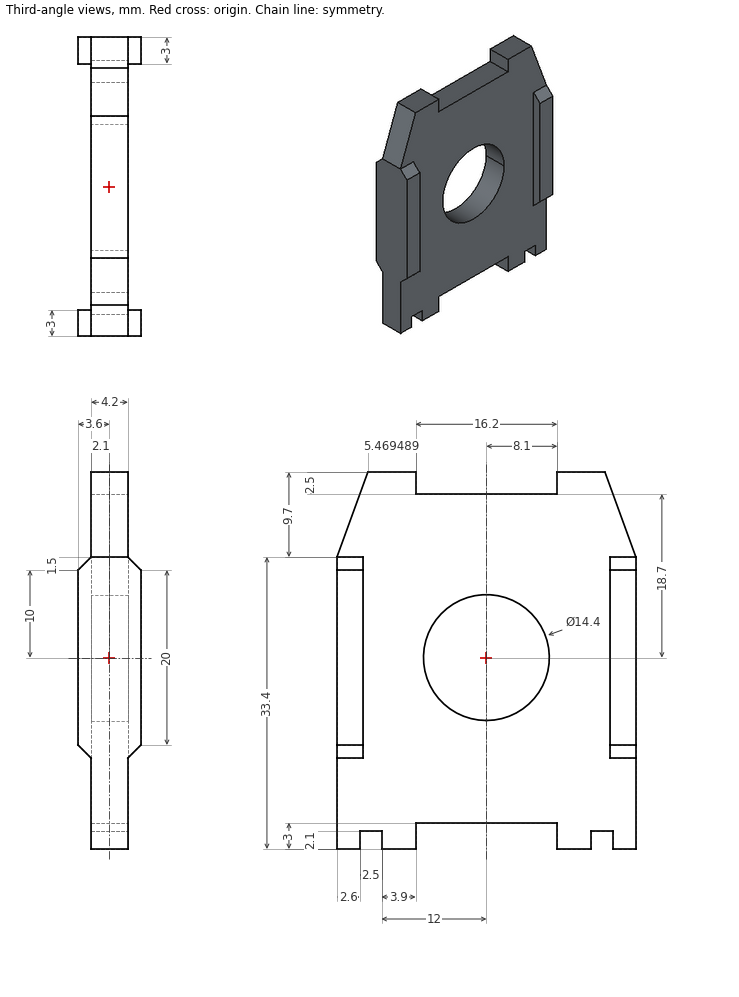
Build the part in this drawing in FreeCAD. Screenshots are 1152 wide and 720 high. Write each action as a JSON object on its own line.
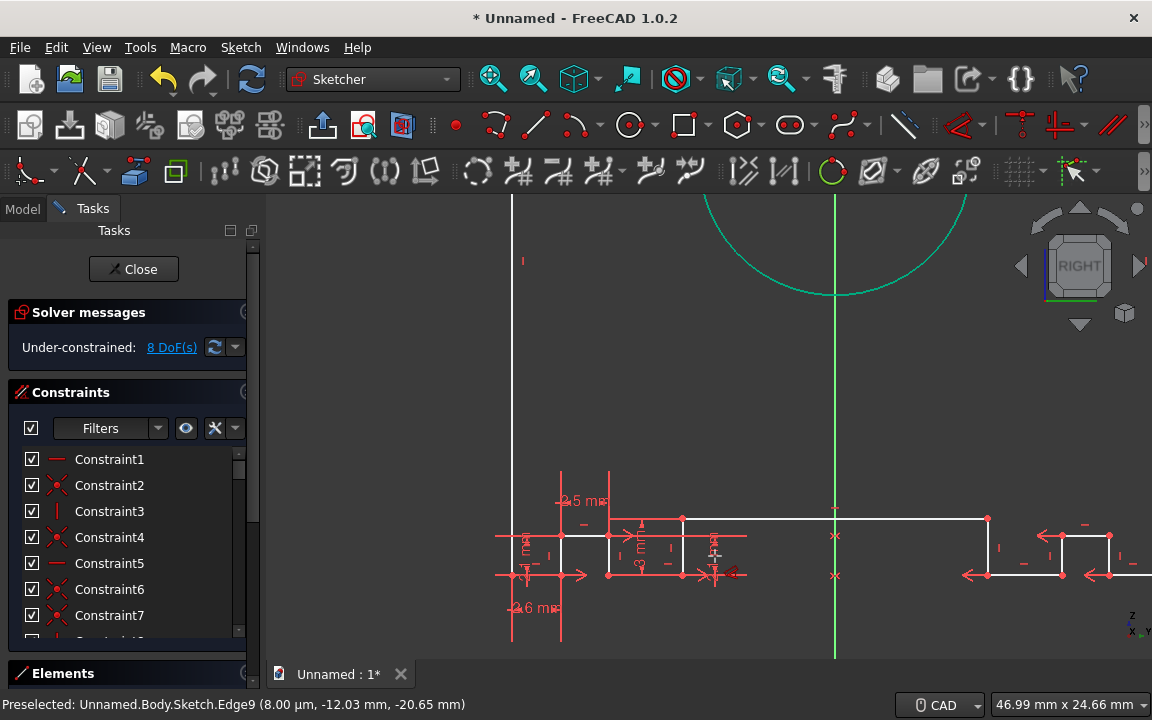
{"action": "left_click", "coordinate": [631, 575]}
{"action": "left_click", "coordinate": [646, 609]}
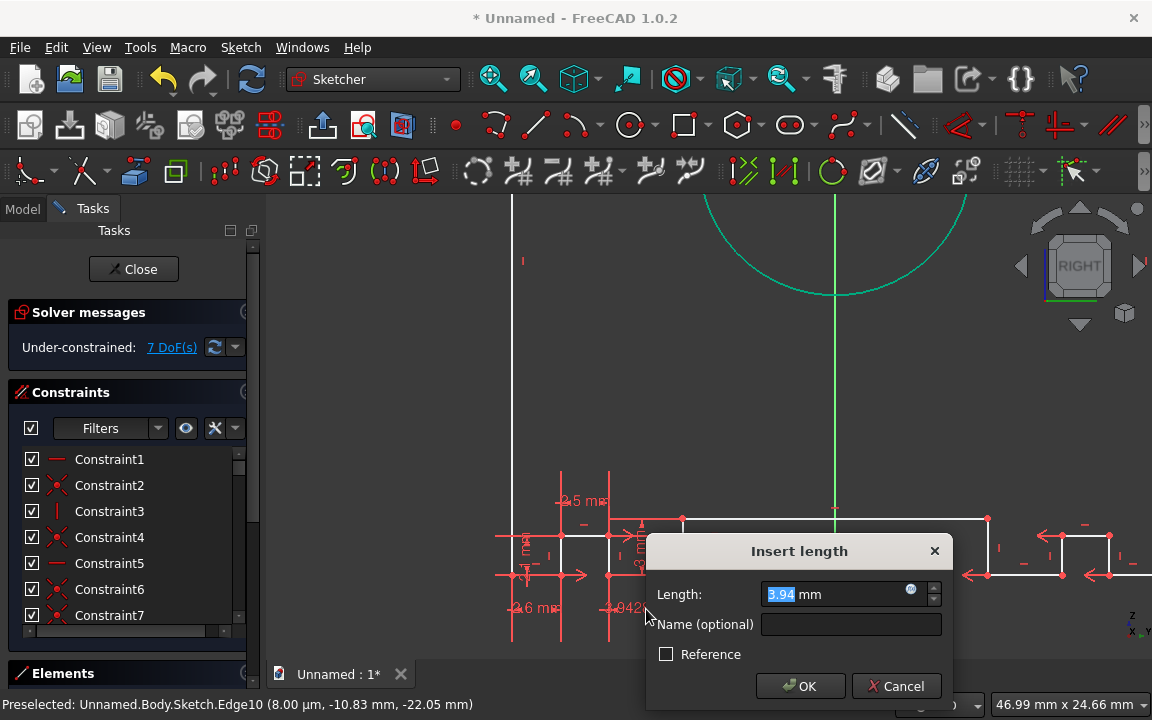
{"action": "type", "text": "3.9"}
{"action": "key", "text": "Return"}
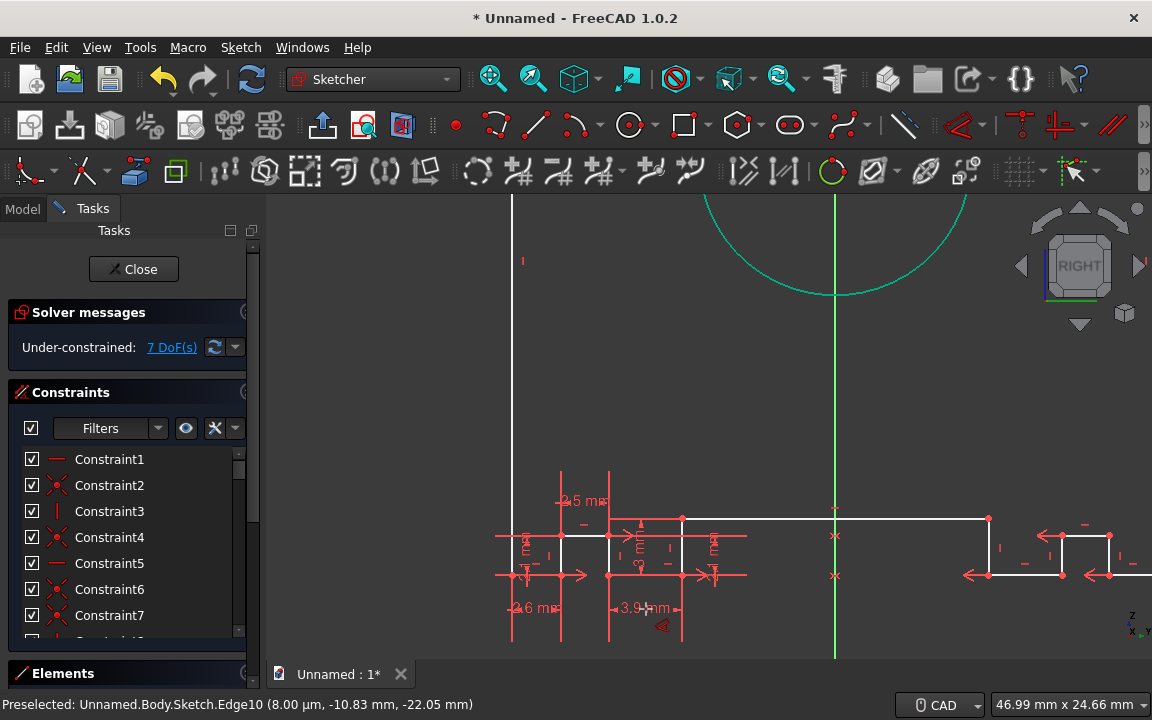
{"action": "left_click", "coordinate": [609, 536]}
{"action": "left_click", "coordinate": [801, 570]}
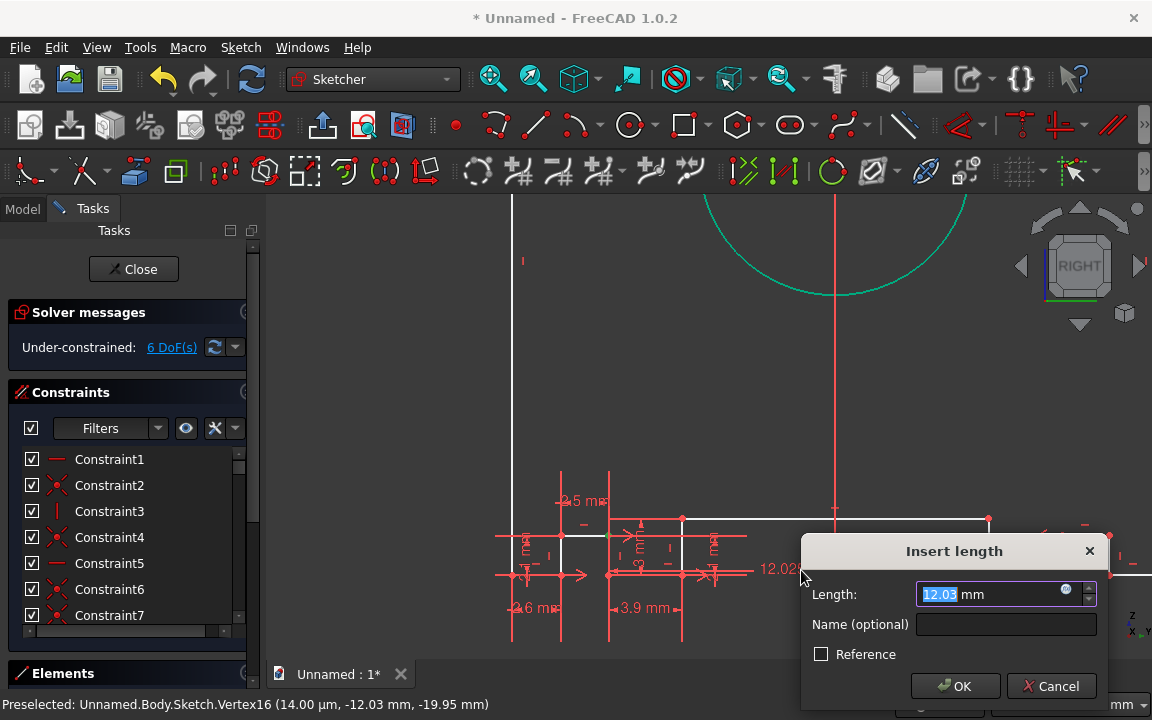
{"action": "type", "text": "12"}
{"action": "key", "text": "Return"}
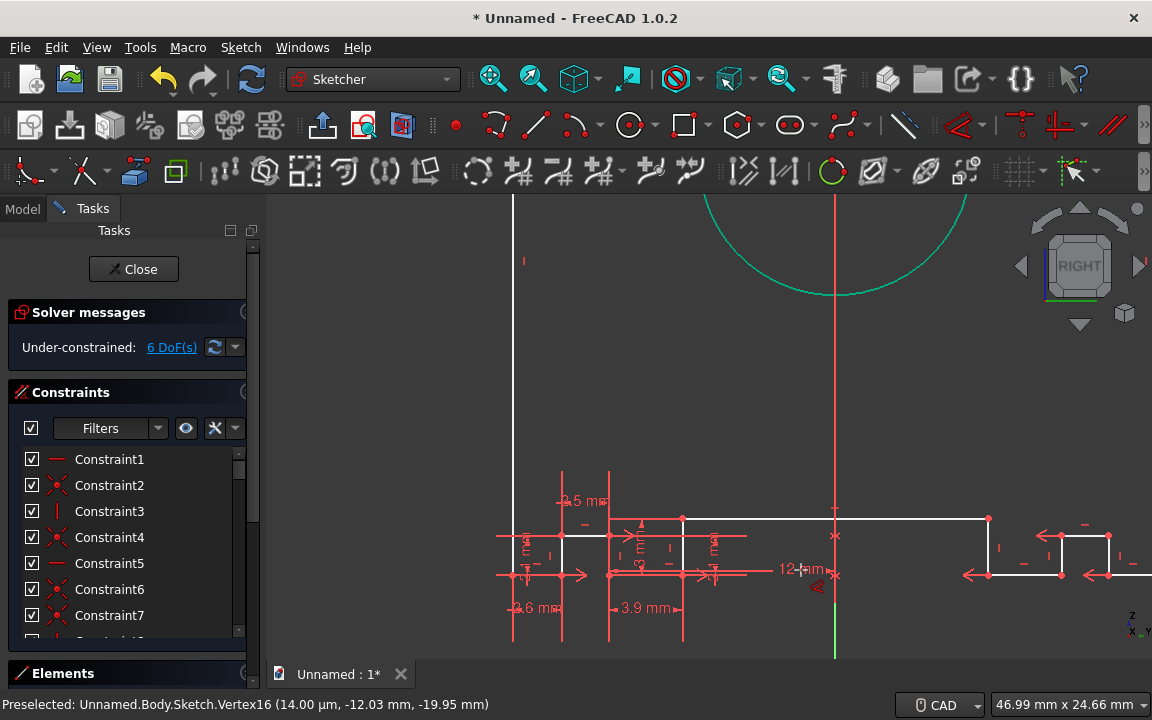
{"action": "scroll", "coordinate": [527, 578], "scroll_direction": "down", "scroll_amount": 5}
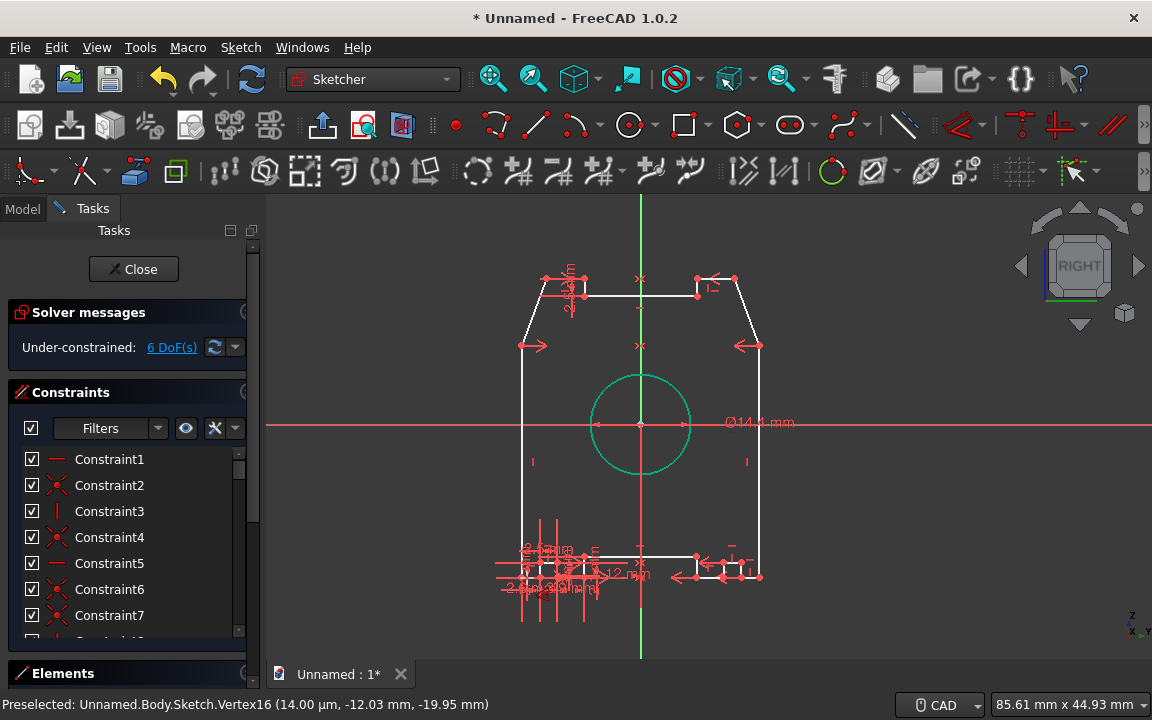
{"action": "left_click", "coordinate": [663, 296]}
{"action": "left_click", "coordinate": [615, 262]}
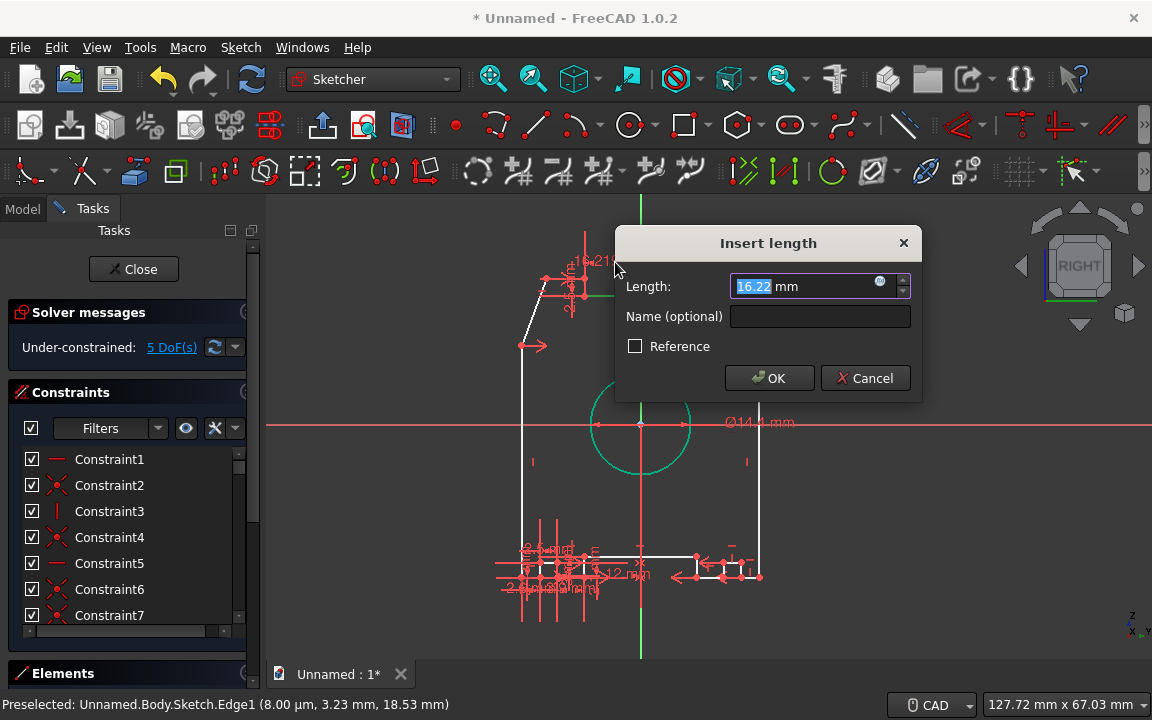
{"action": "type", "text": "16.2"}
{"action": "key", "text": "Return"}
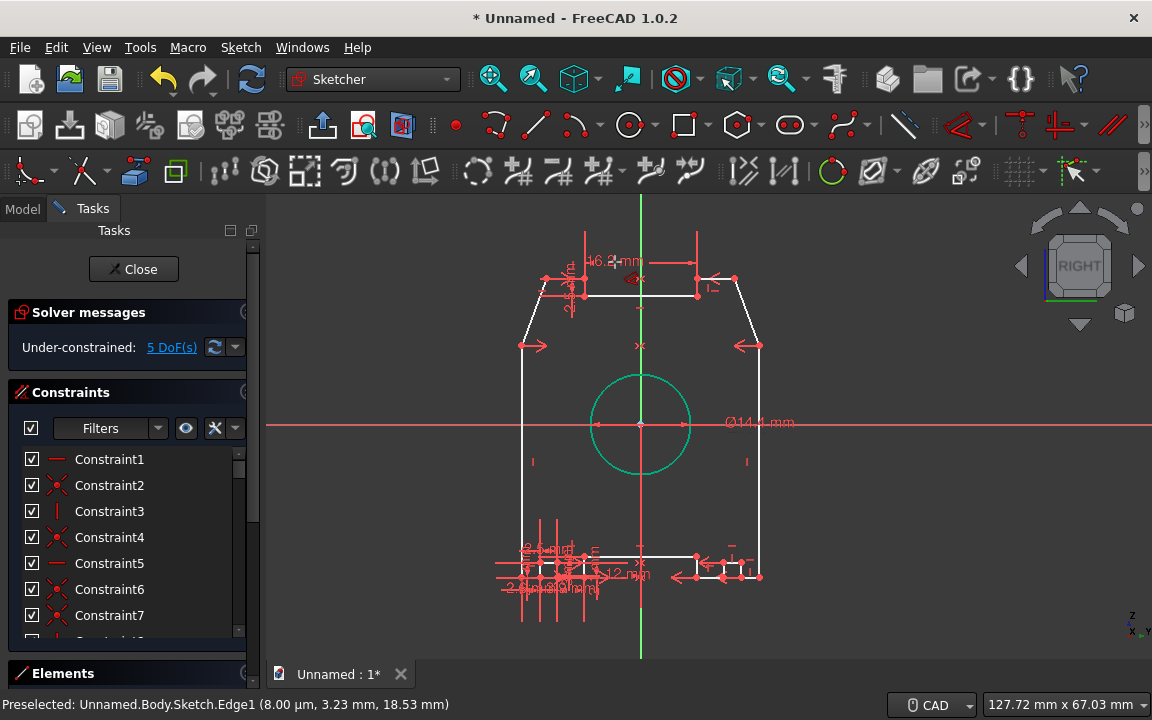
{"action": "scroll", "coordinate": [522, 415], "scroll_direction": "up", "scroll_amount": 3}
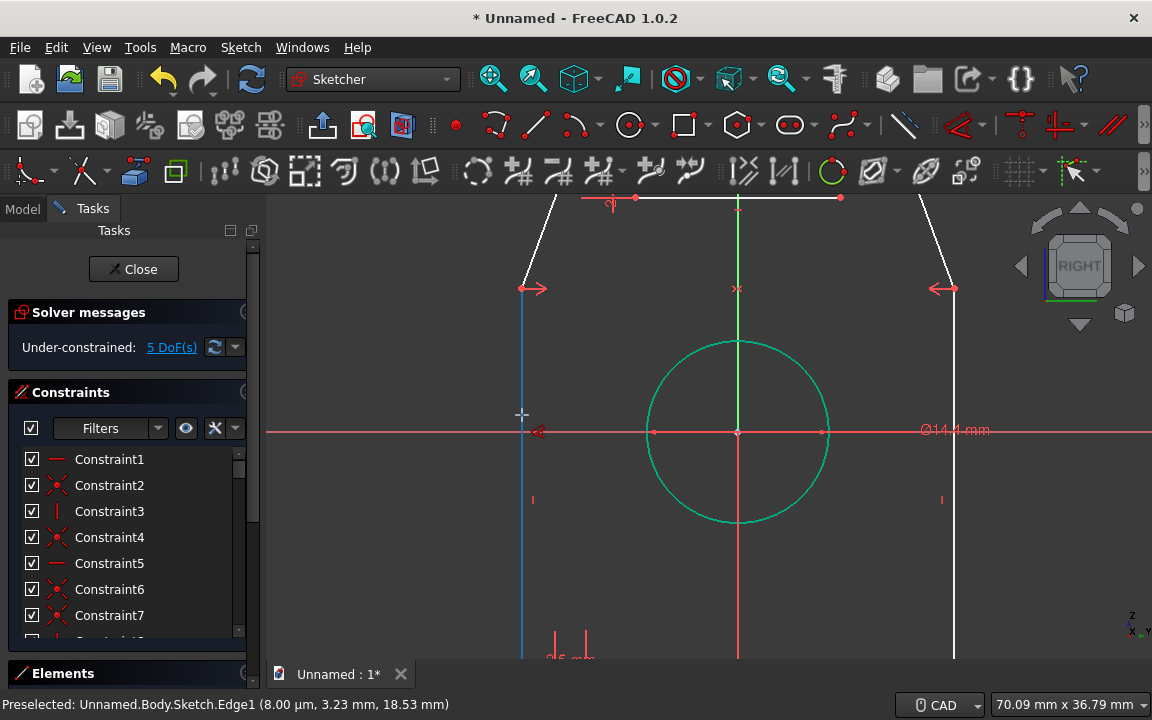
{"action": "left_click", "coordinate": [522, 415]}
{"action": "left_click", "coordinate": [488, 460]}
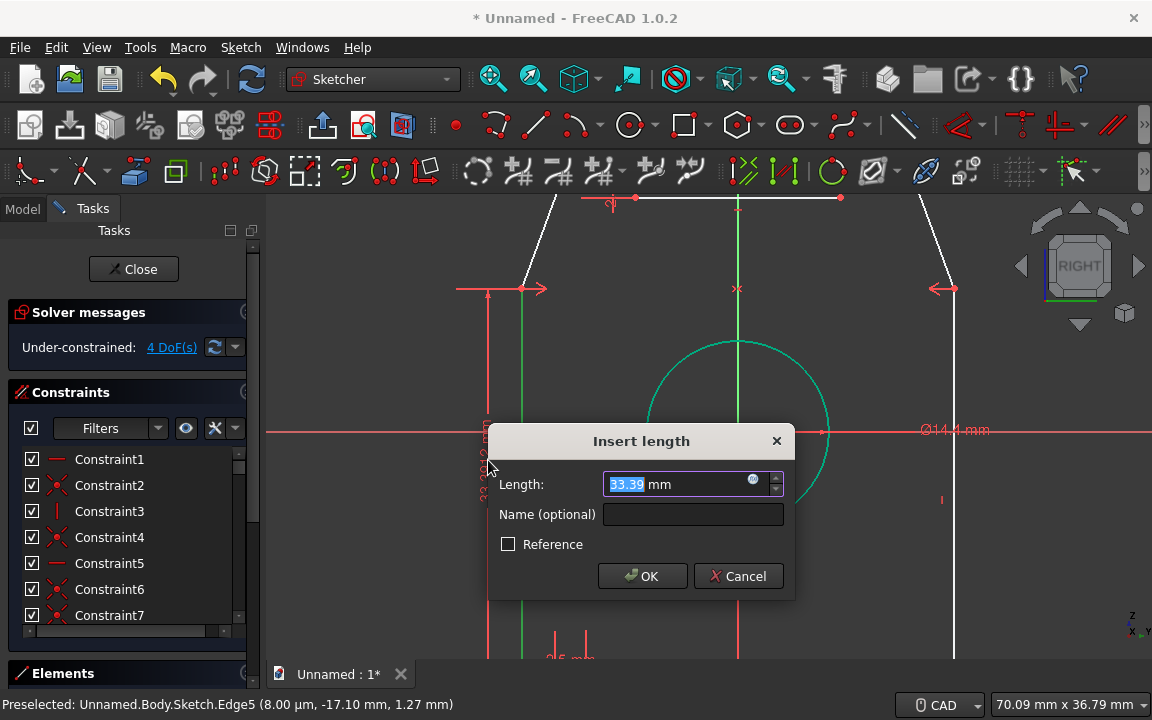
{"action": "type", "text": "33.4"}
{"action": "key", "text": "Return"}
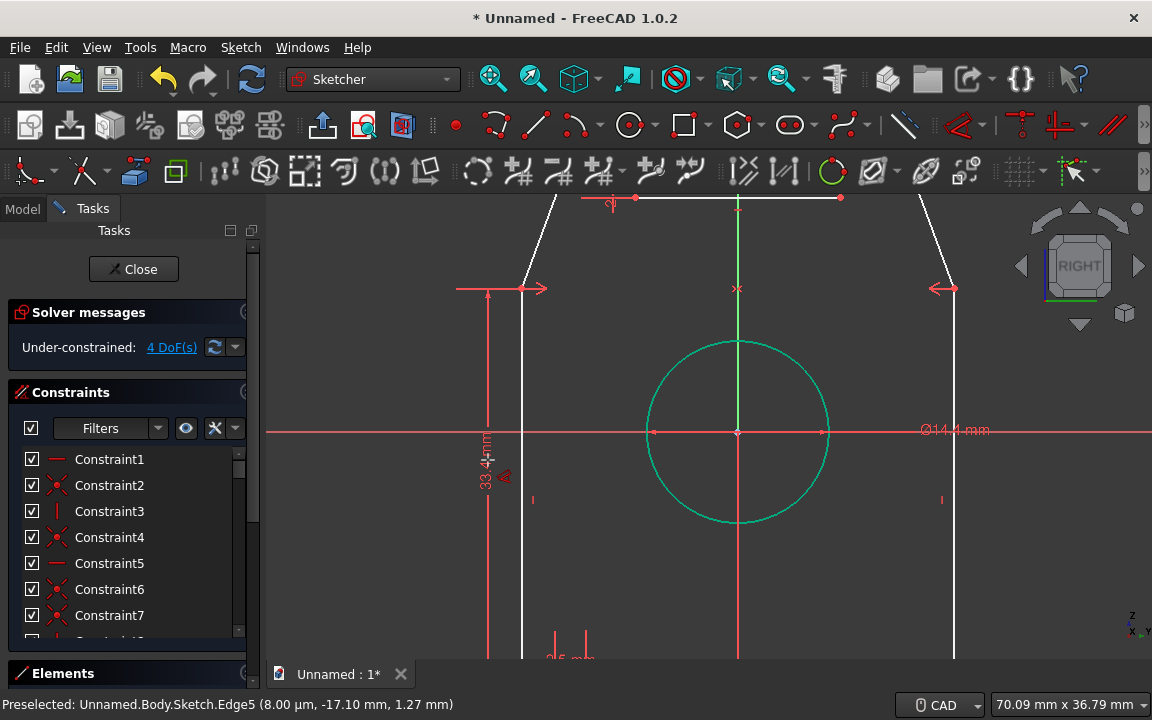
{"action": "scroll", "coordinate": [522, 414], "scroll_direction": "down", "scroll_amount": 3}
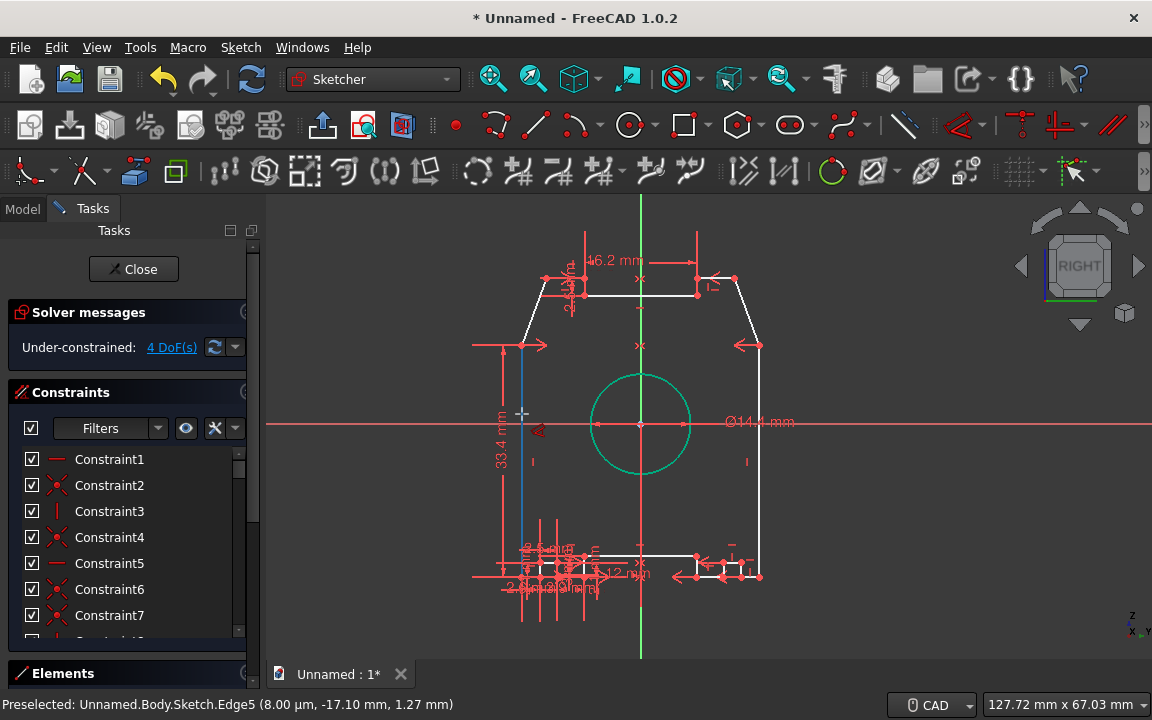
{"action": "left_click", "coordinate": [697, 296]}
{"action": "left_click", "coordinate": [689, 262]}